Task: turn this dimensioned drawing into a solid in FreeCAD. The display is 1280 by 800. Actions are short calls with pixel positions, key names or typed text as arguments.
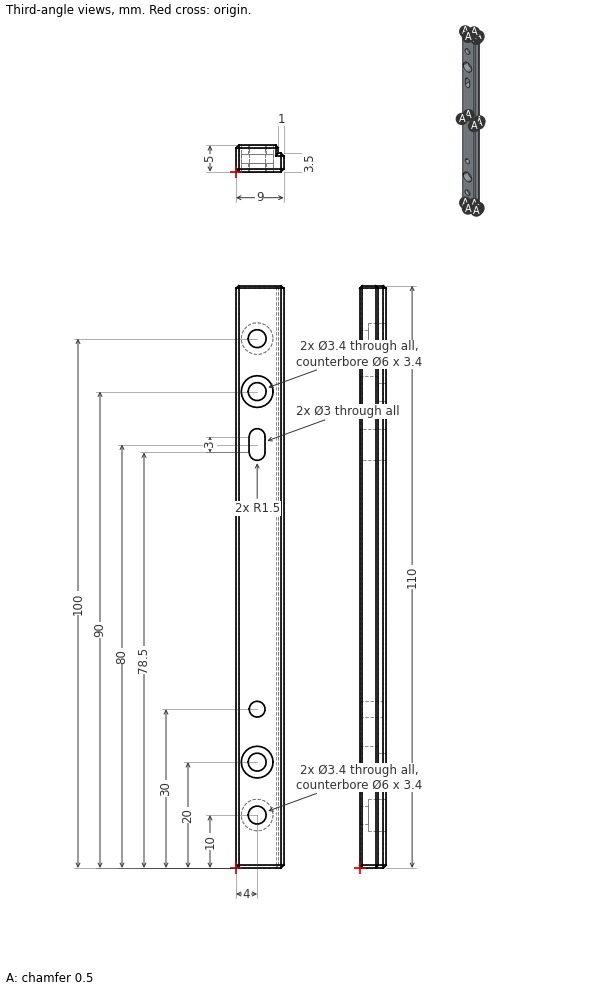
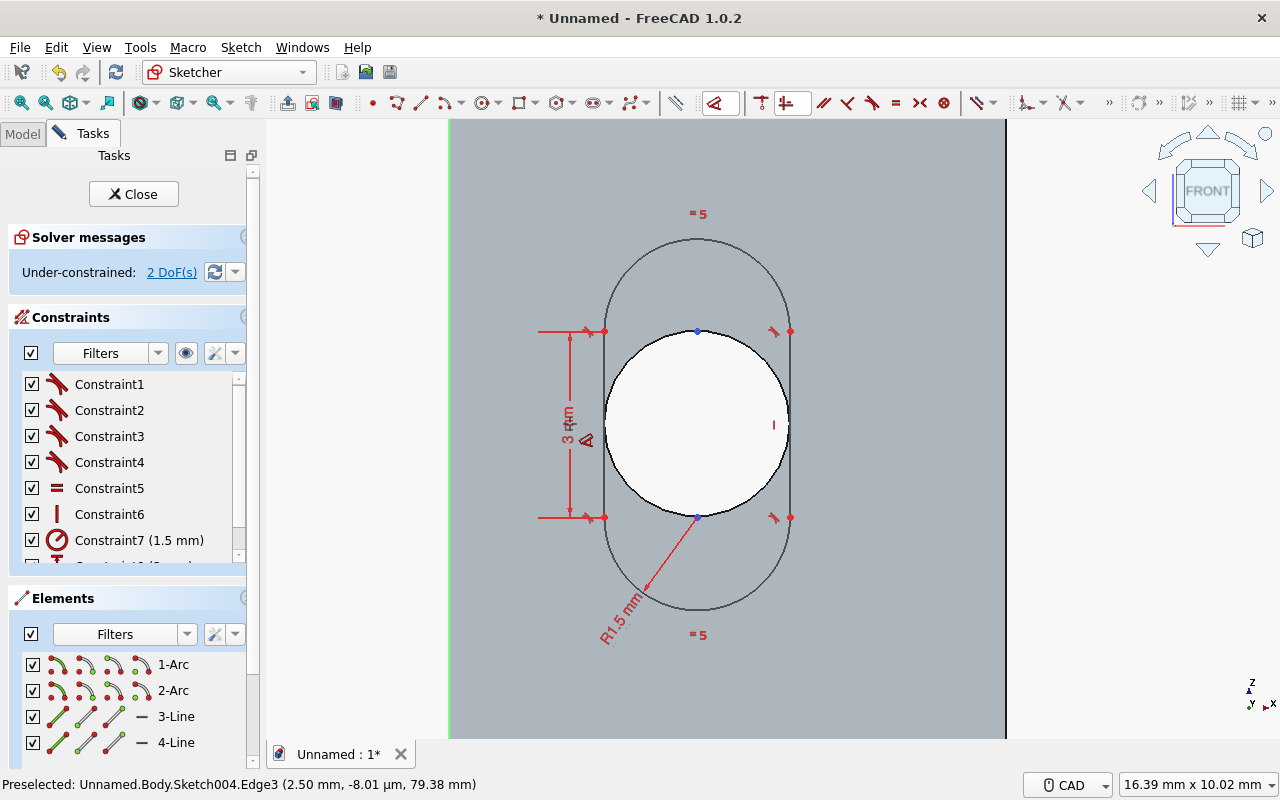
click(697, 518)
click(573, 484)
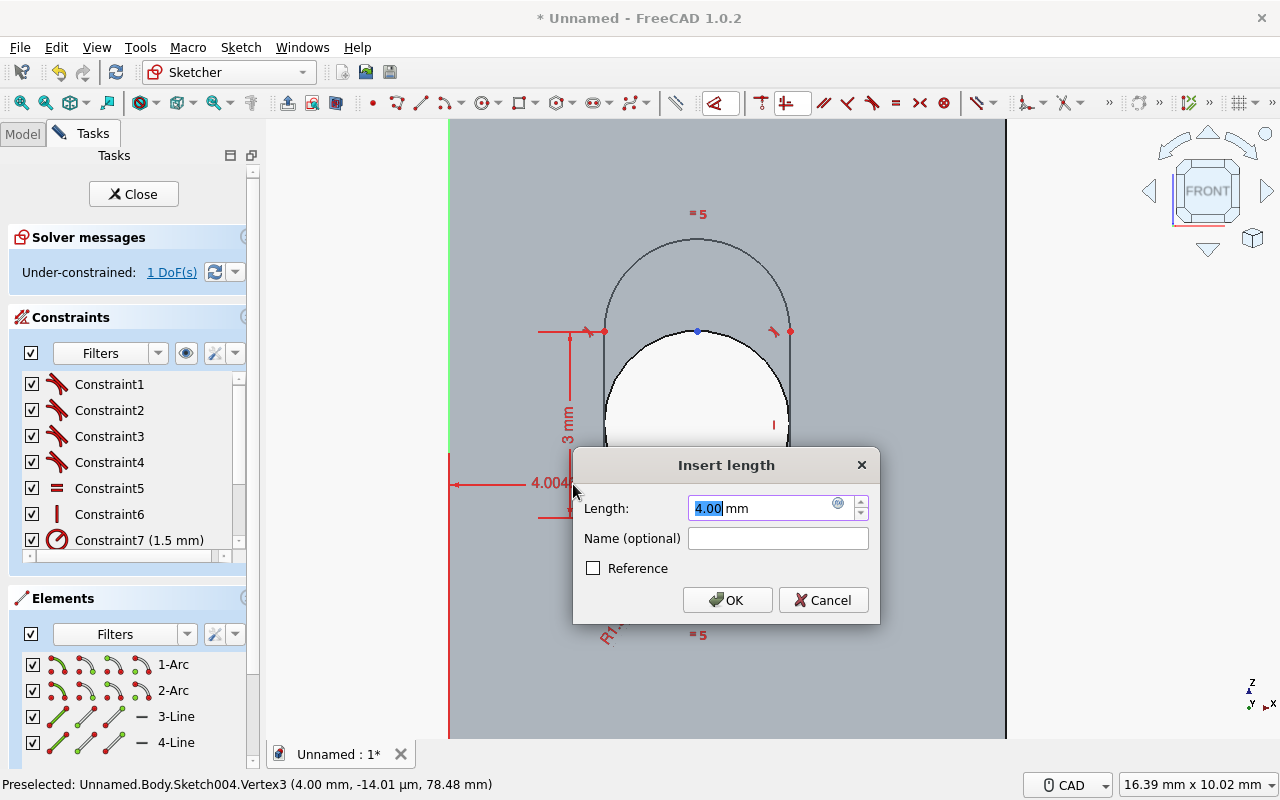
text(4)
key(Return)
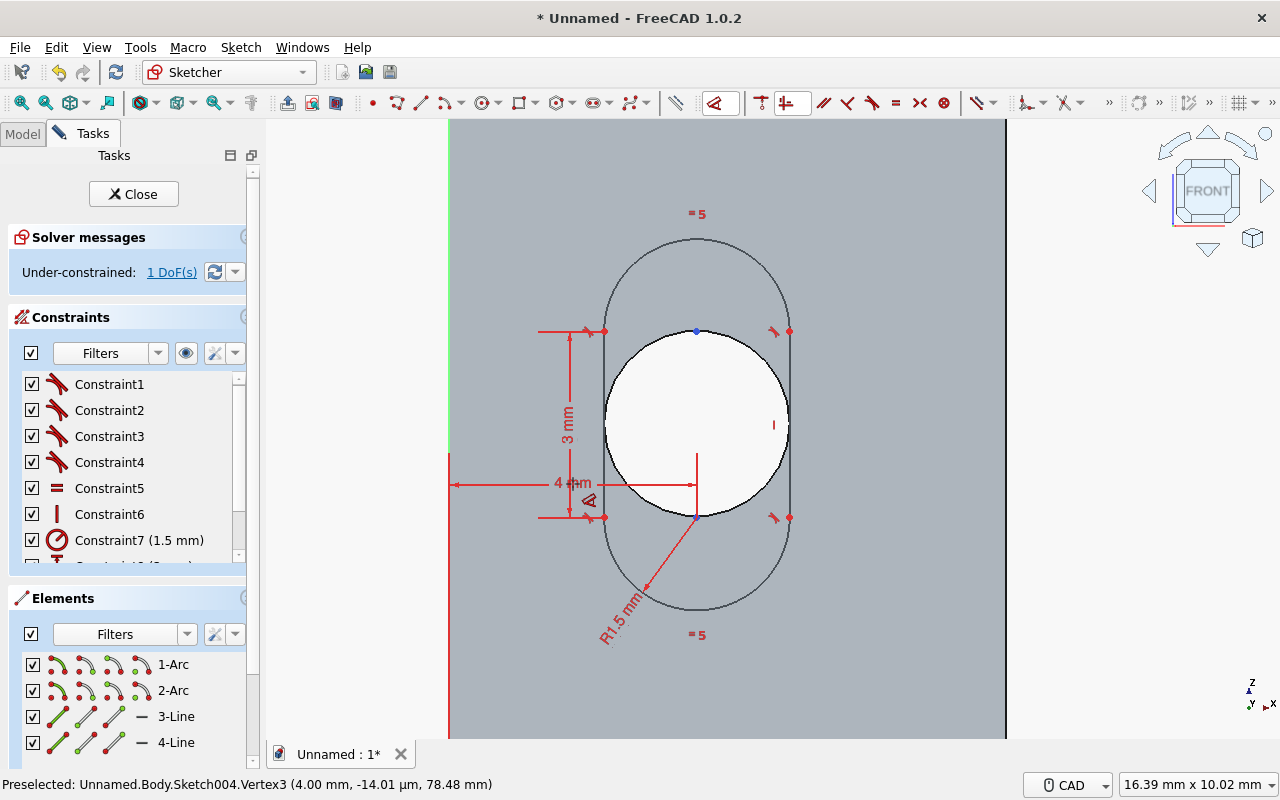
click(604, 518)
click(415, 614)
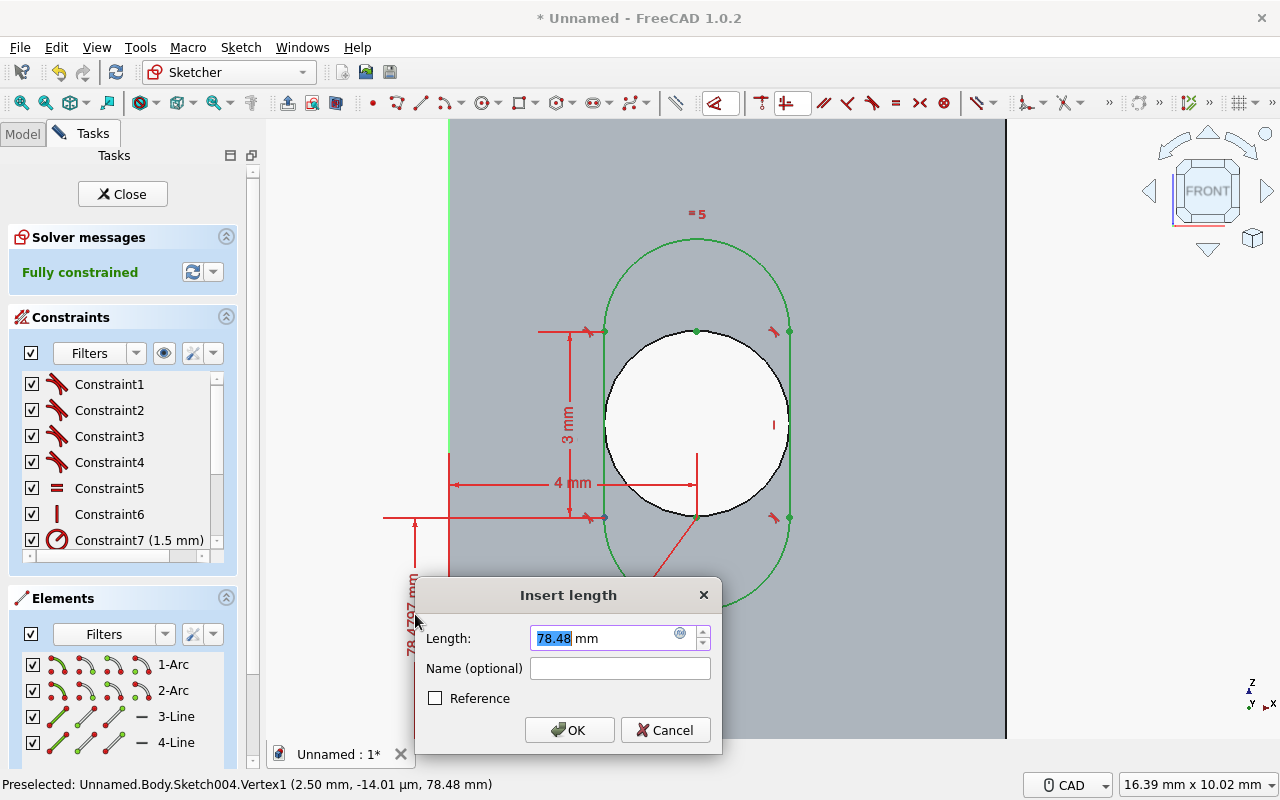
text(78.5)
key(Return)
key(Escape)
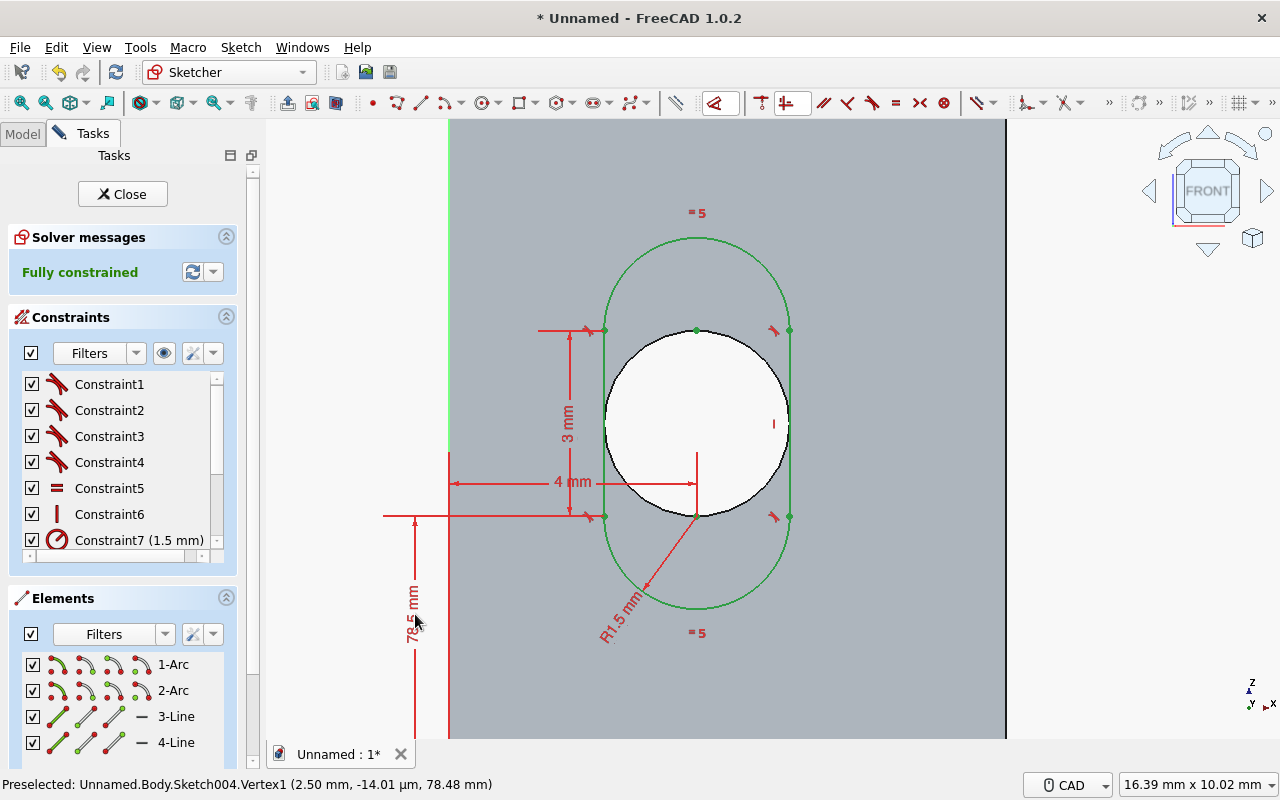
click(123, 194)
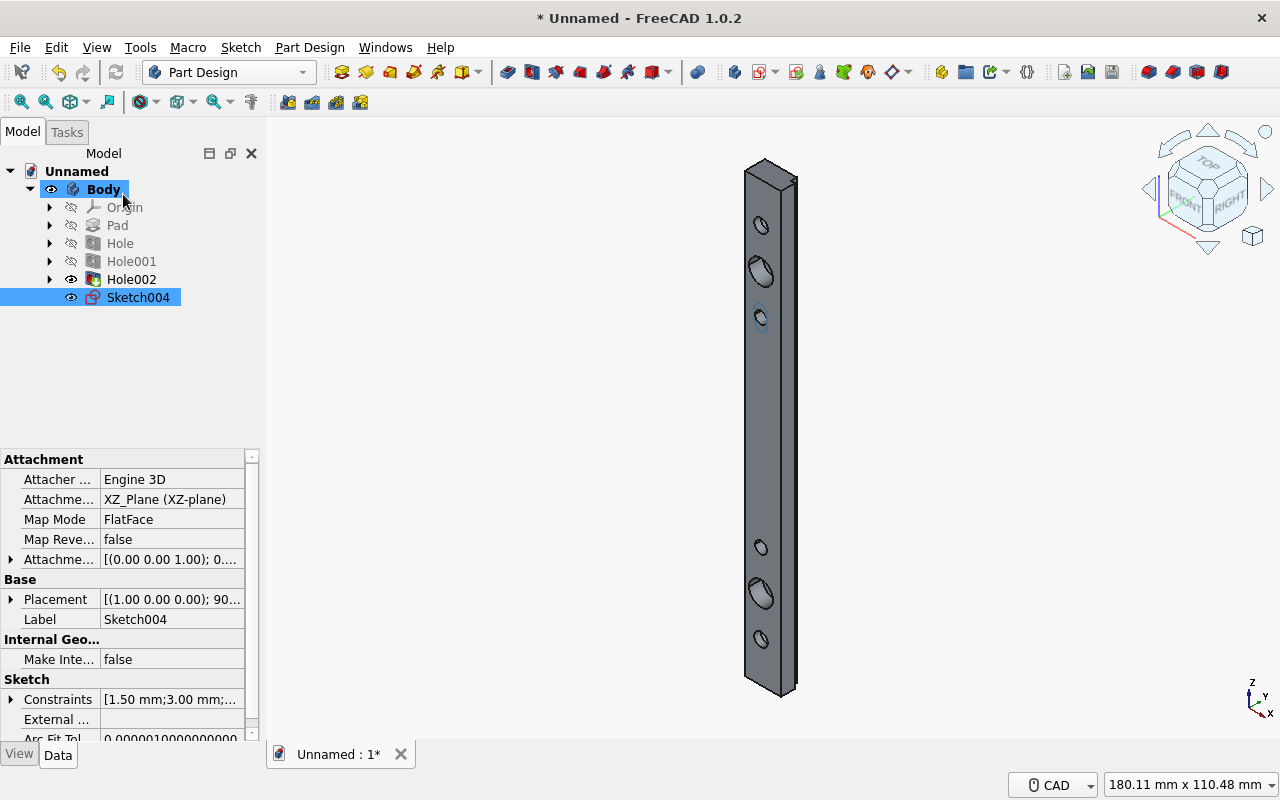
click(508, 72)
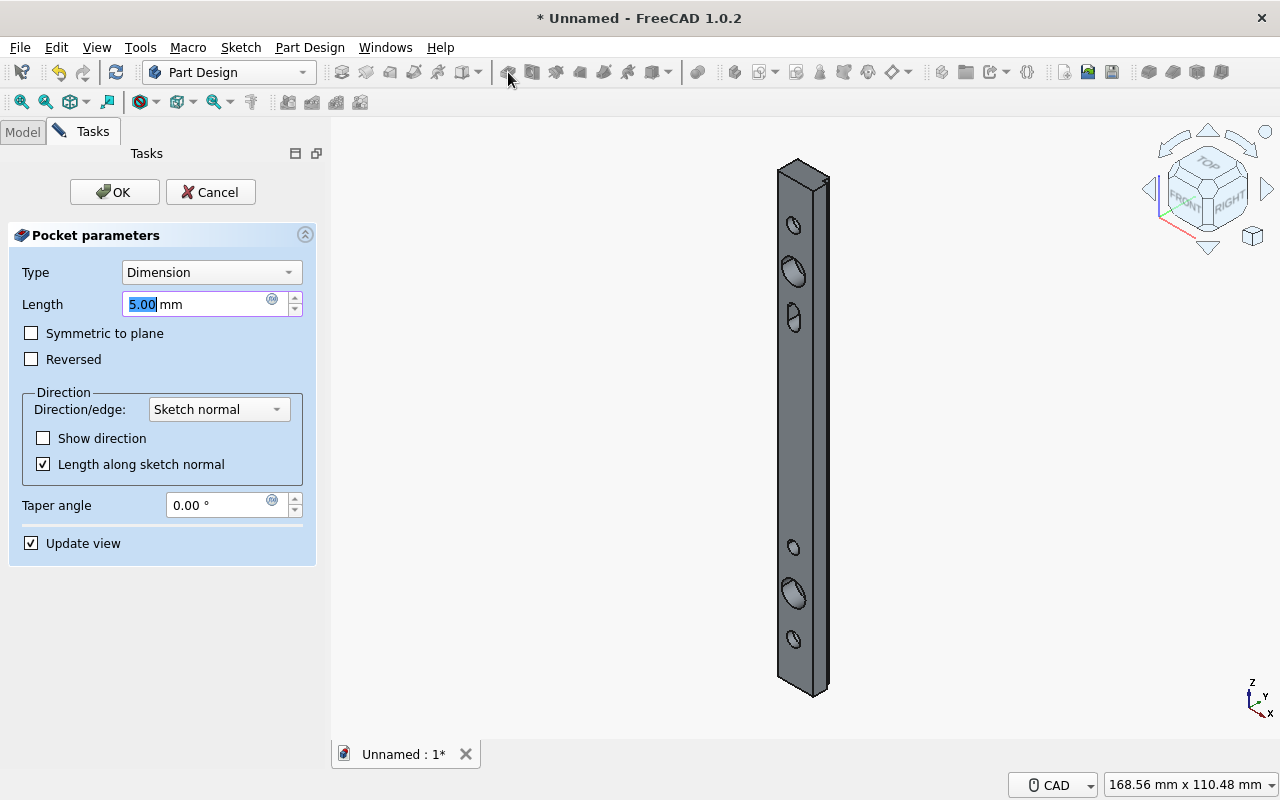
click(212, 272)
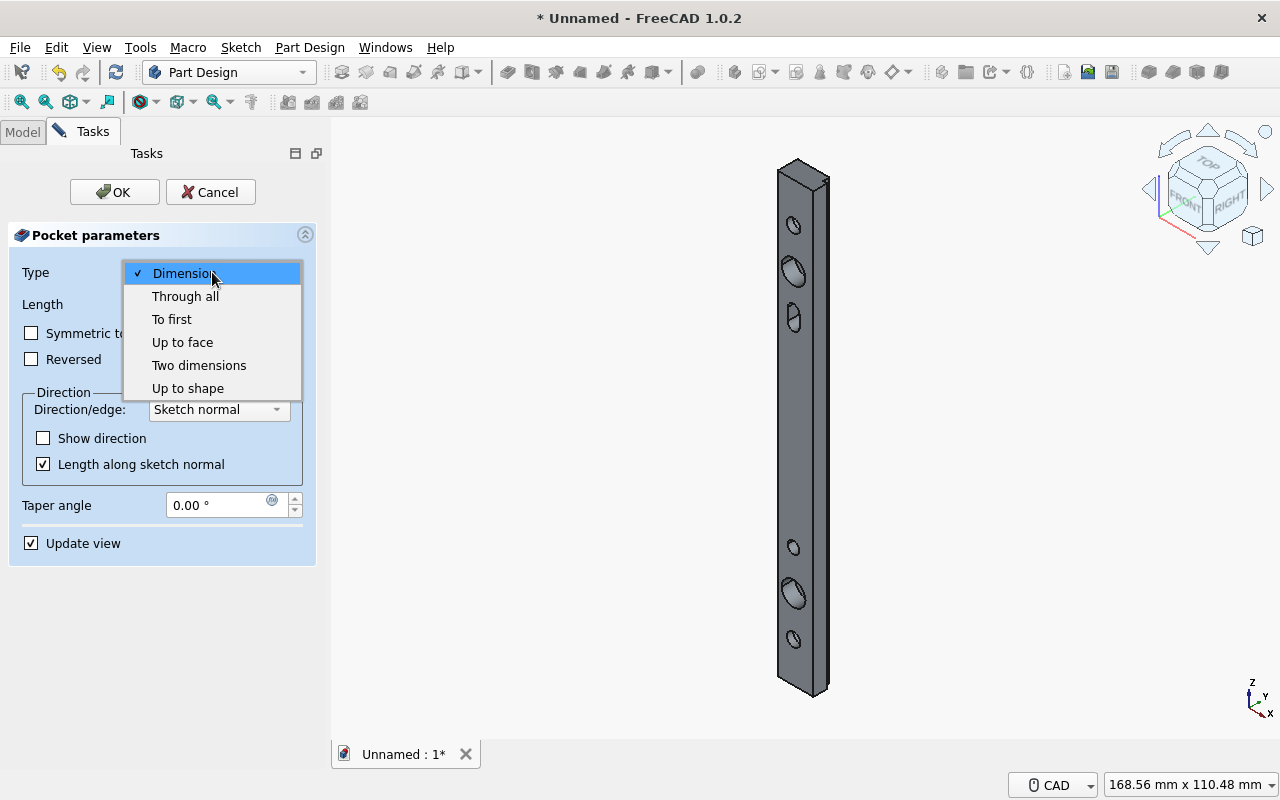
click(212, 296)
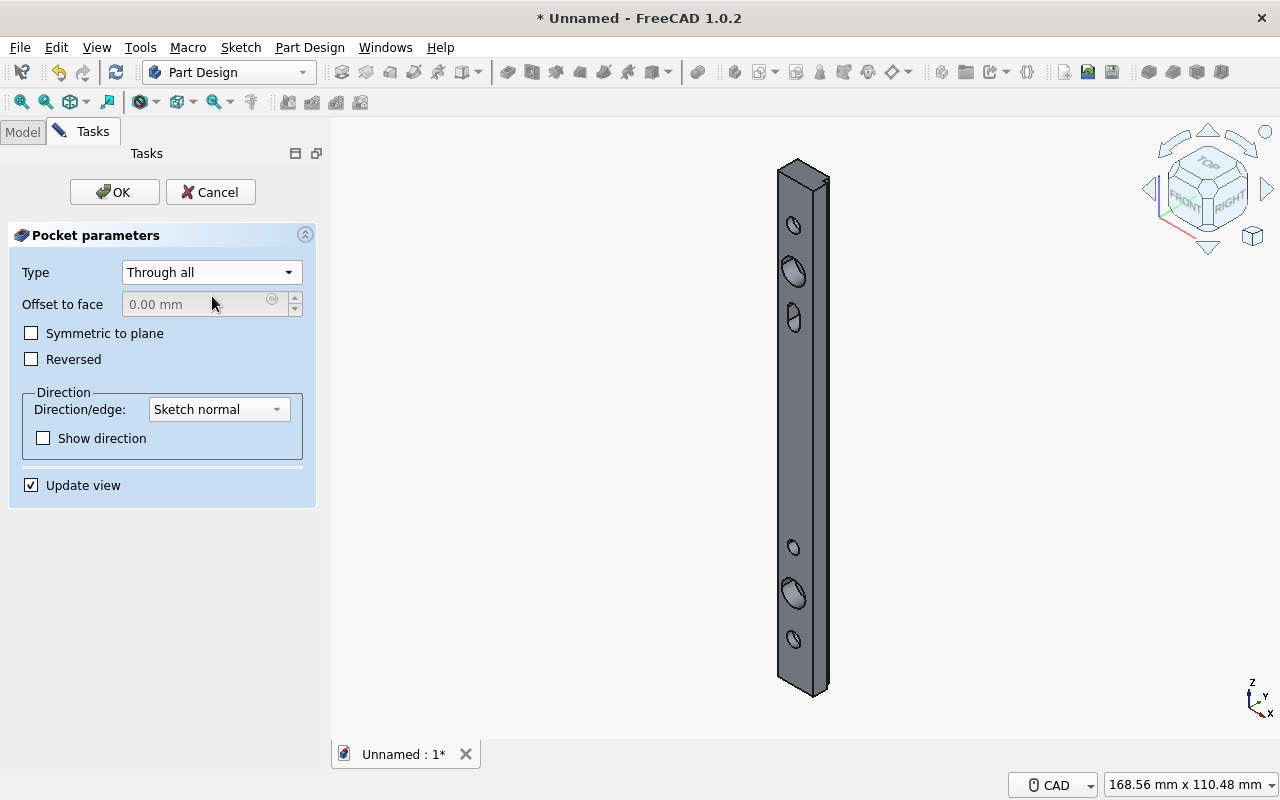
click(115, 192)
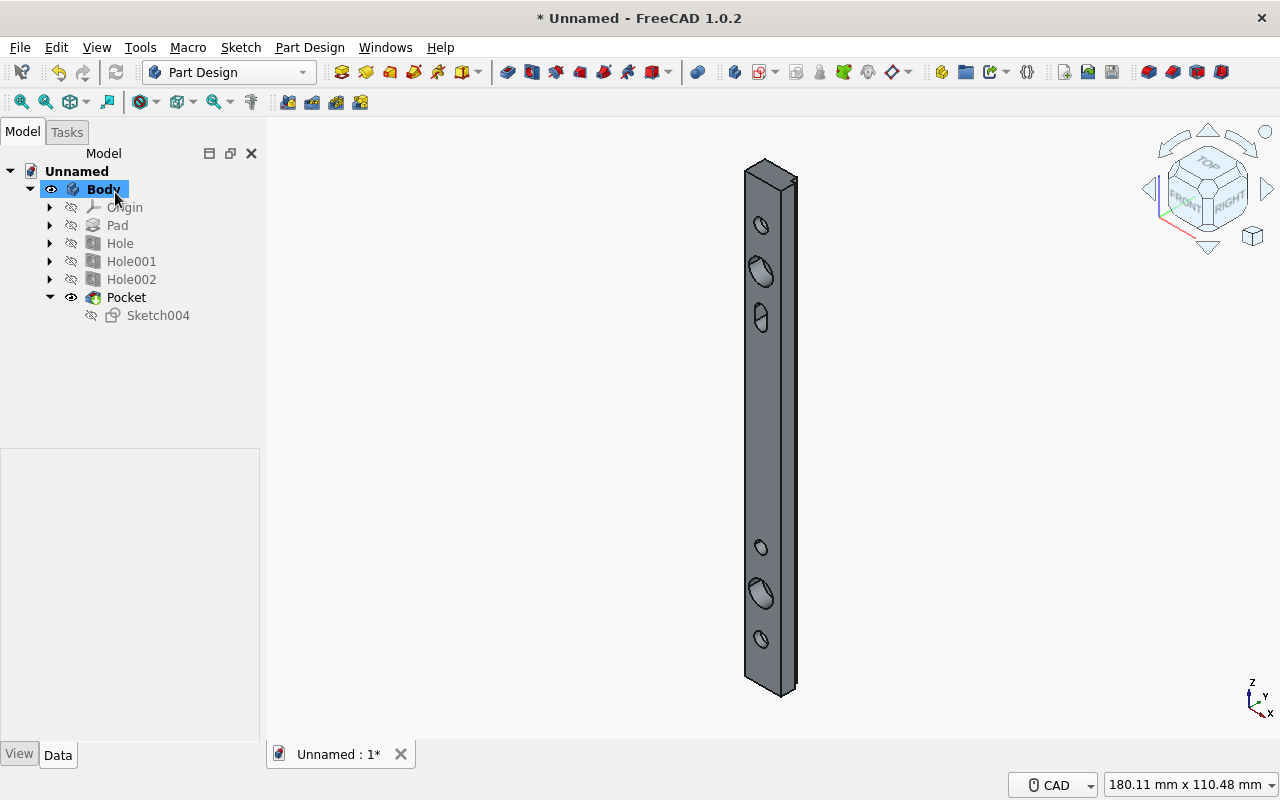
click(790, 221)